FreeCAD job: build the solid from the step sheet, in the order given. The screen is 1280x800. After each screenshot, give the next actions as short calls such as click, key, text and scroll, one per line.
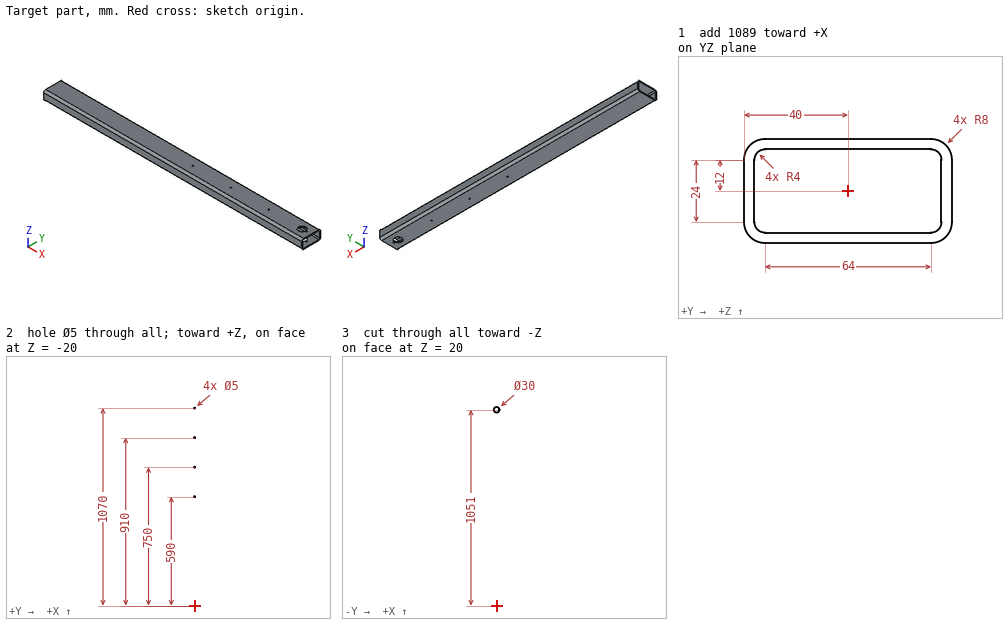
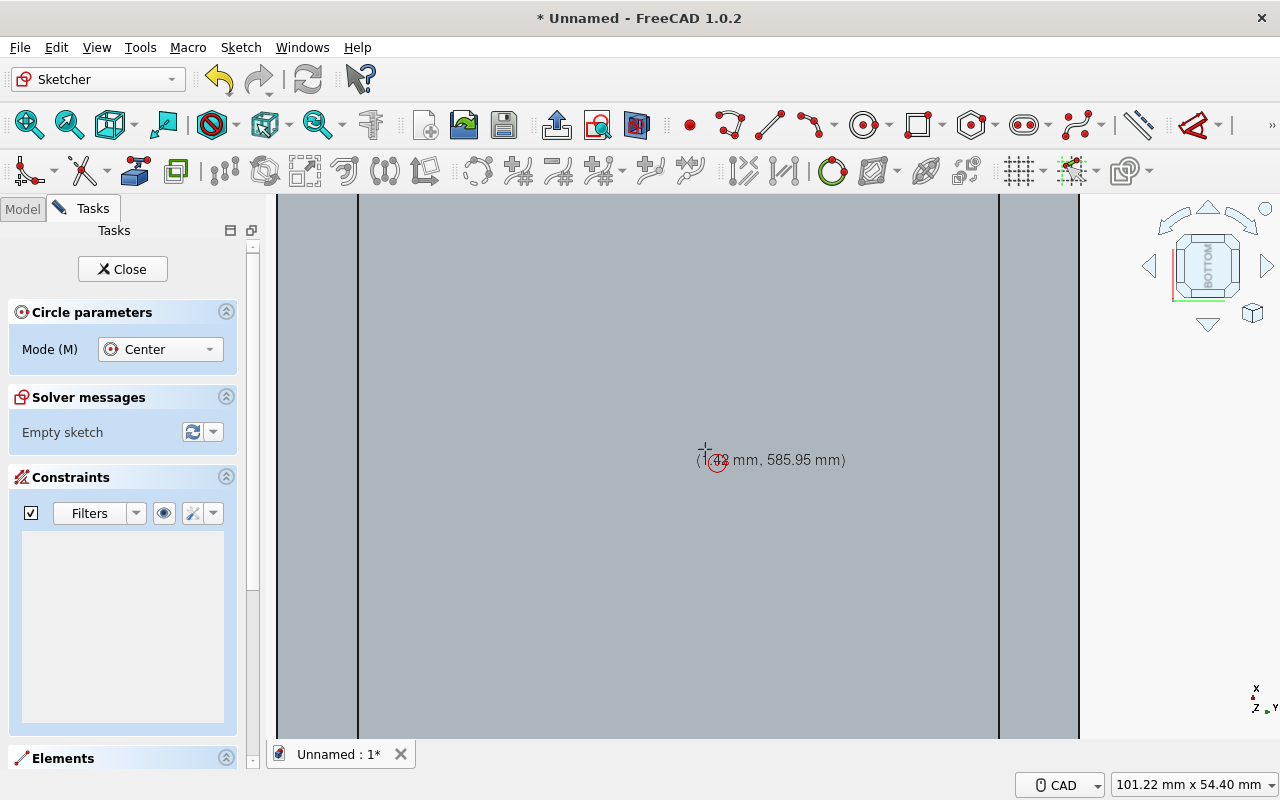
scroll(706, 445, down, 16)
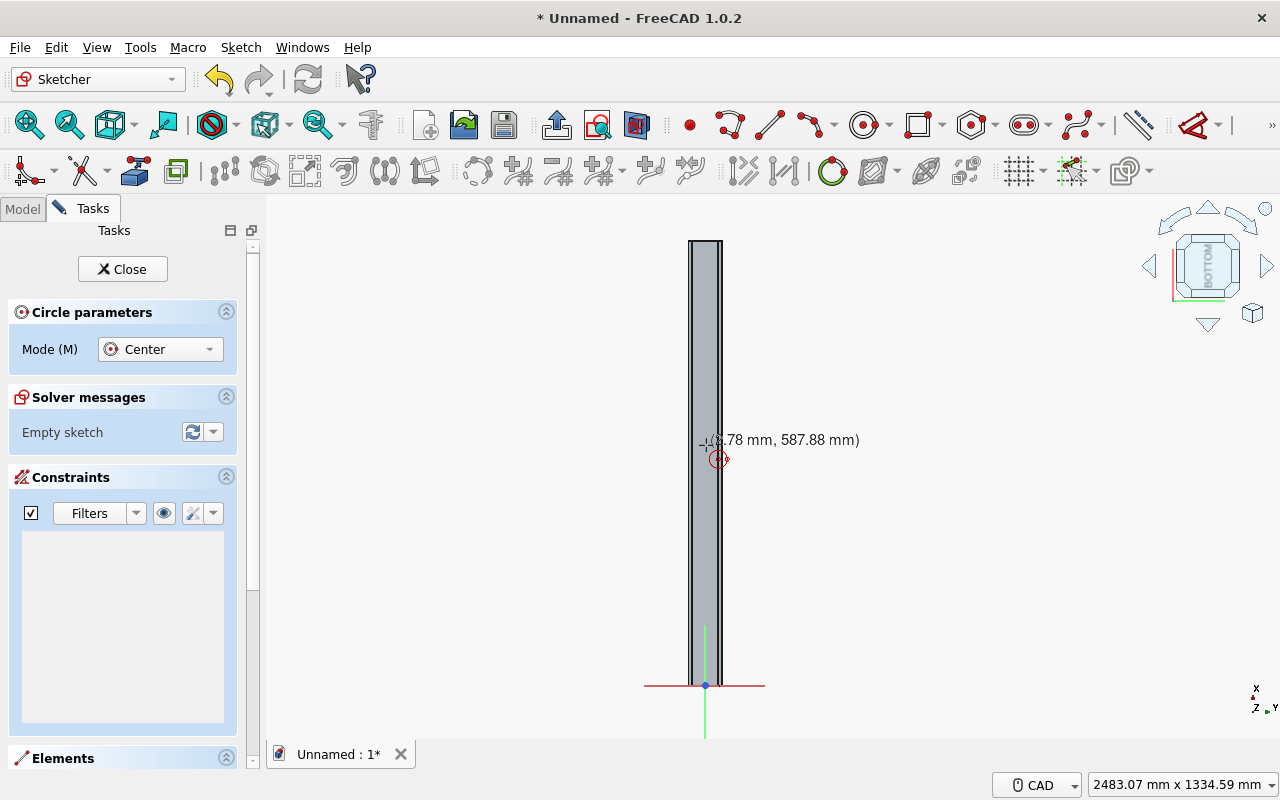
click(705, 445)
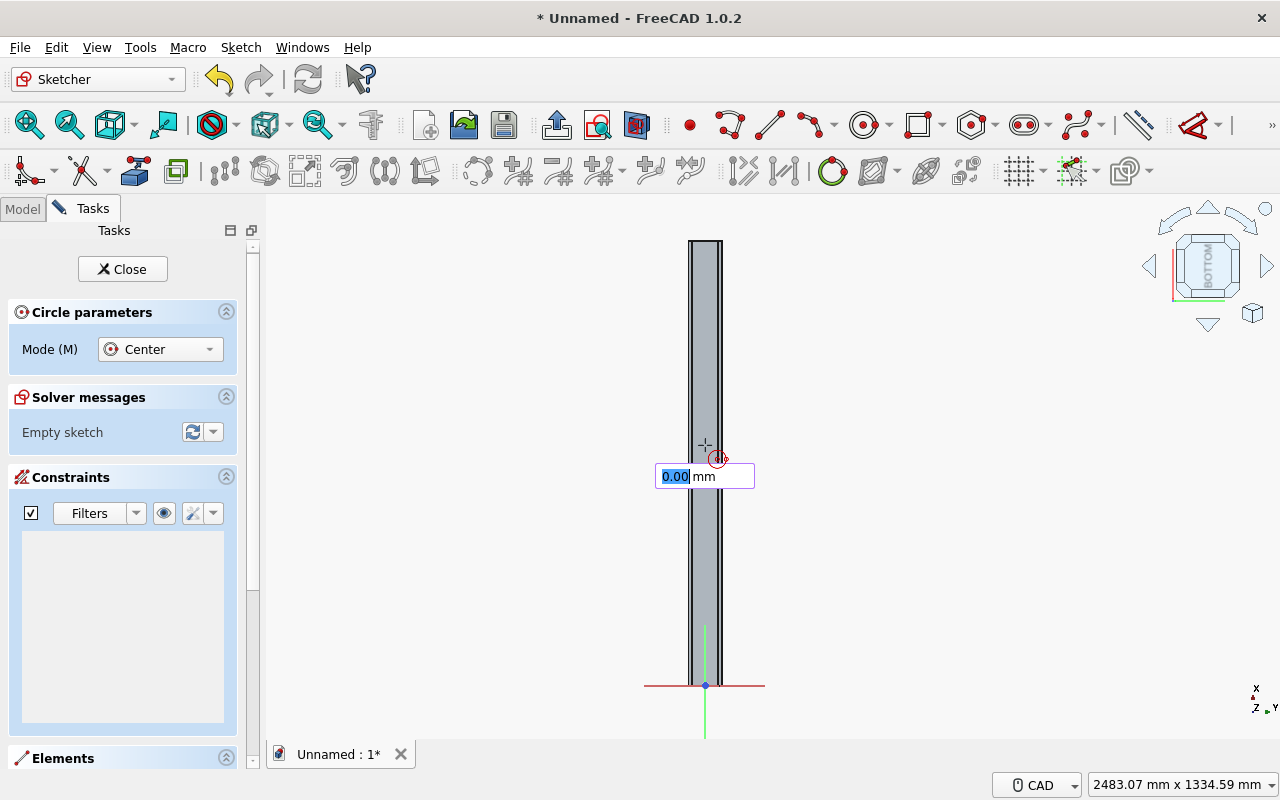
scroll(706, 444, up, 15)
move(703, 441)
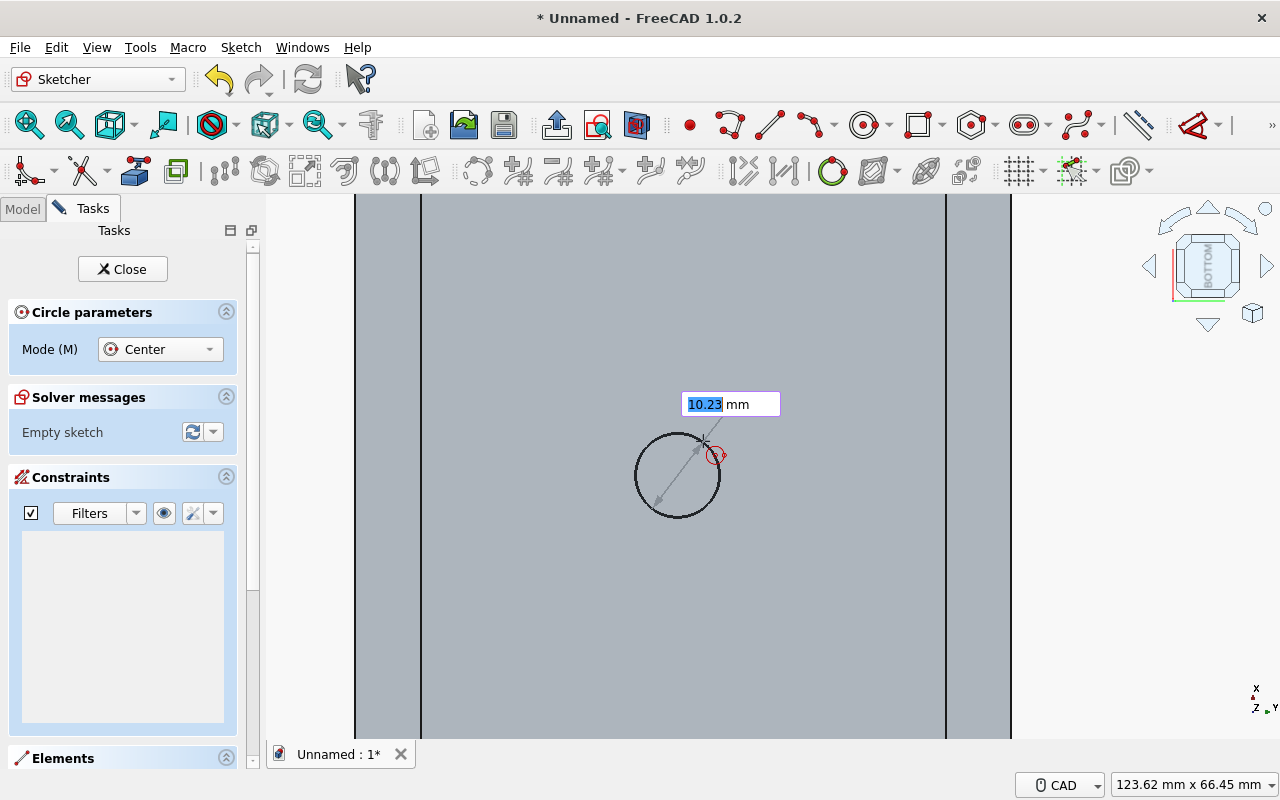
text(5)
key(Return)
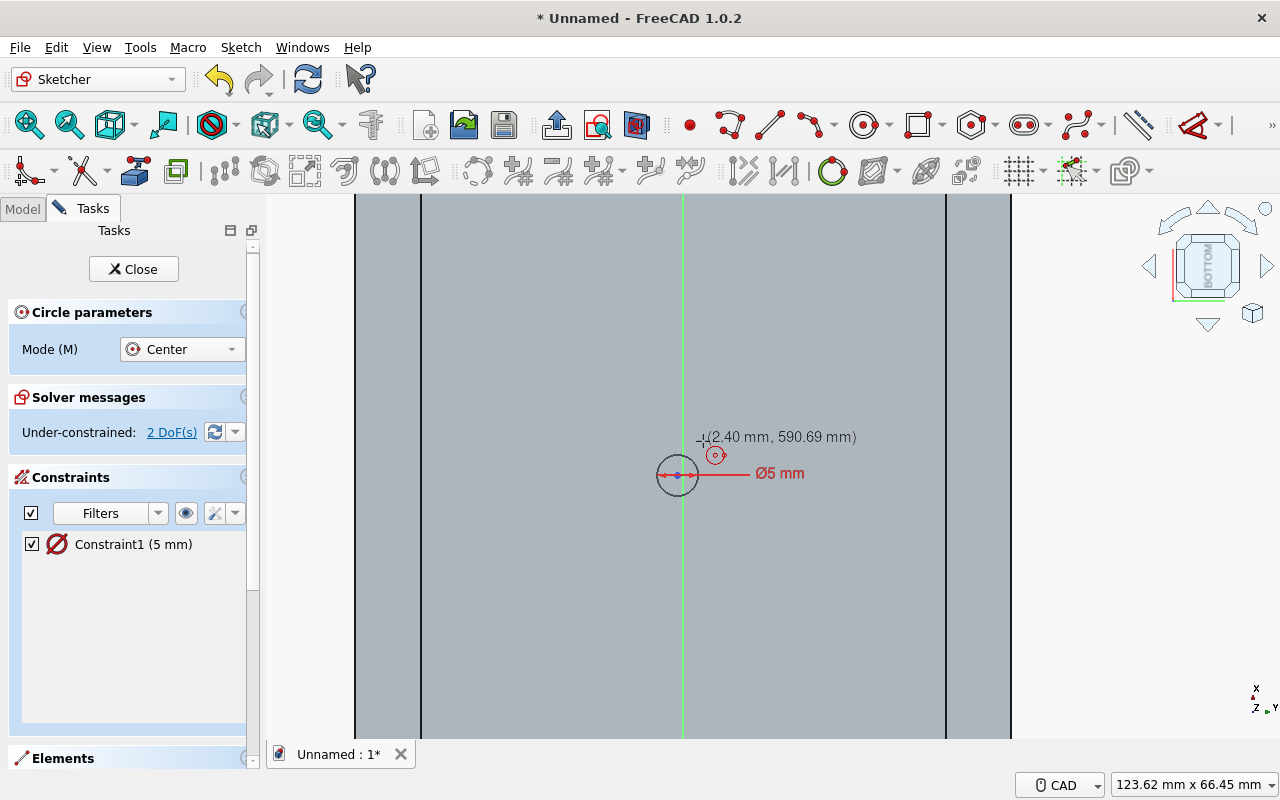
scroll(706, 444, down, 15)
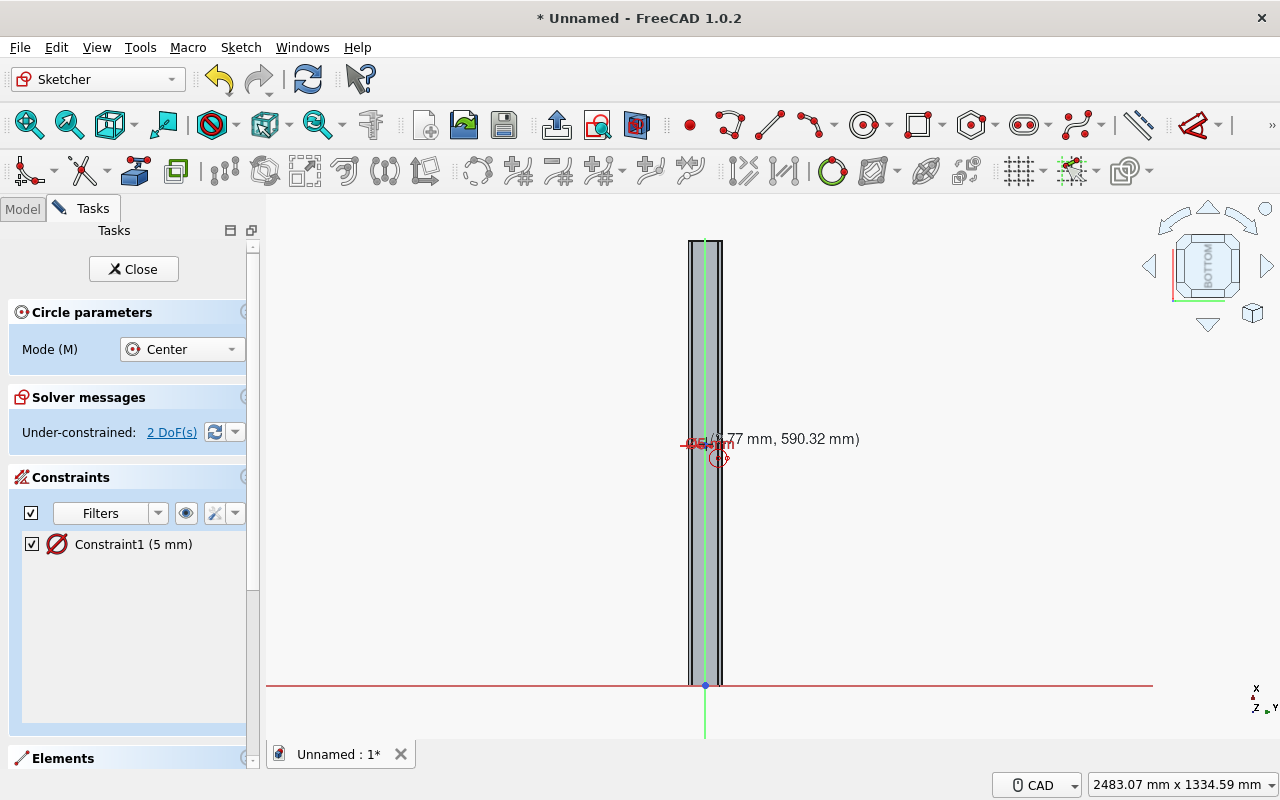
scroll(705, 379, up, 16)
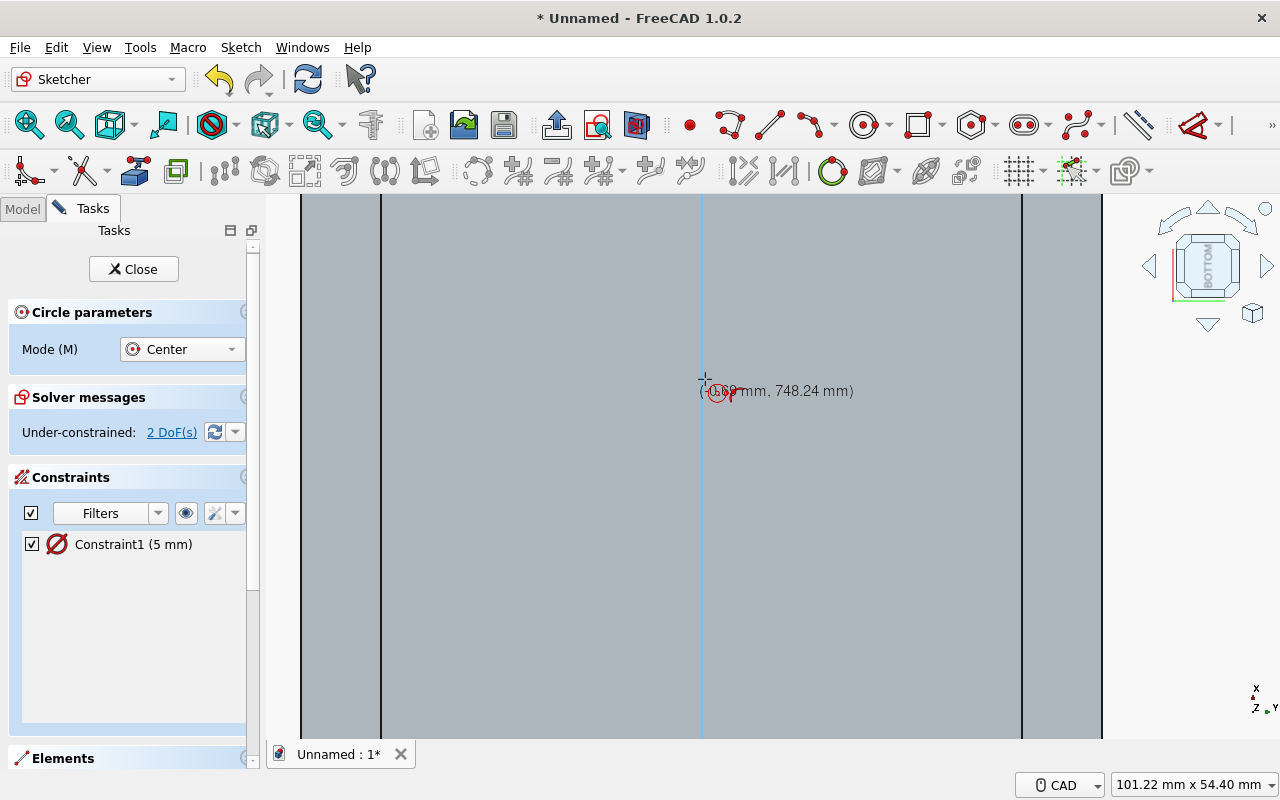
scroll(705, 379, down, 16)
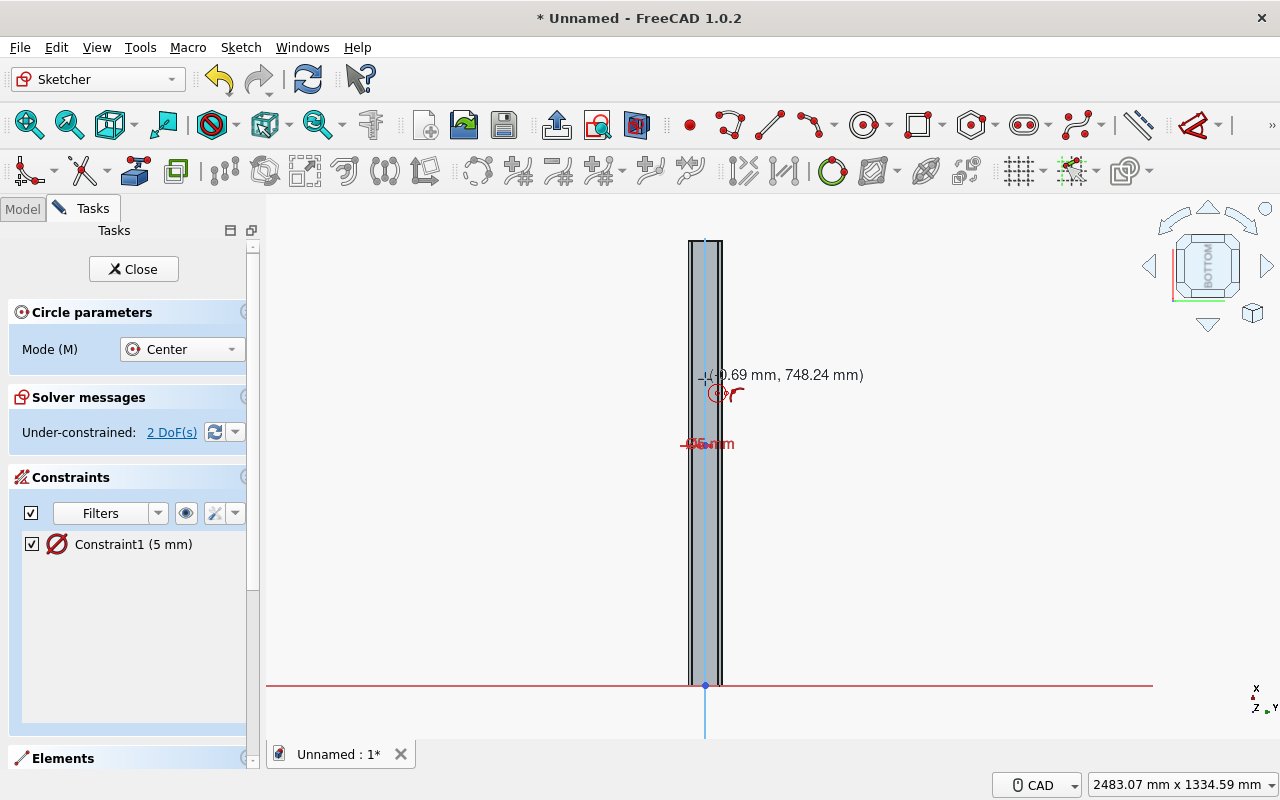
click(705, 379)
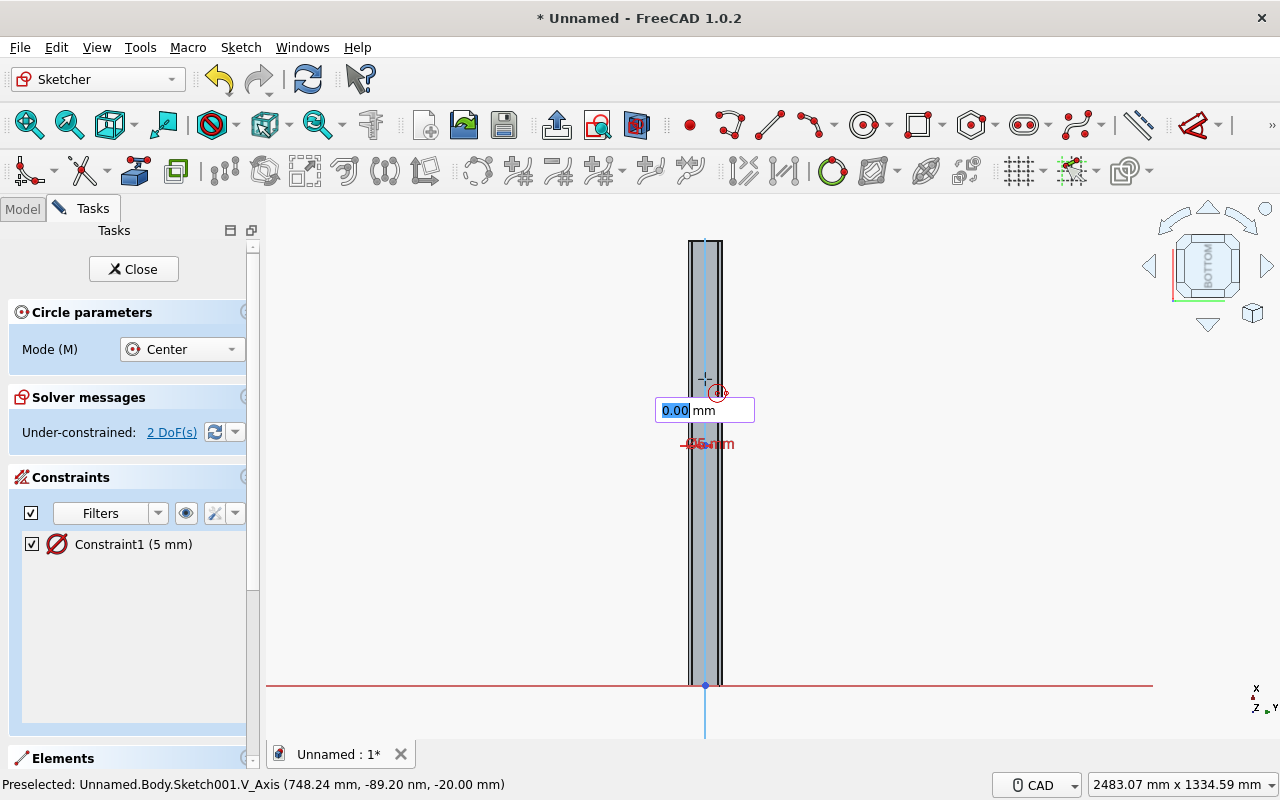
scroll(706, 379, up, 15)
move(703, 371)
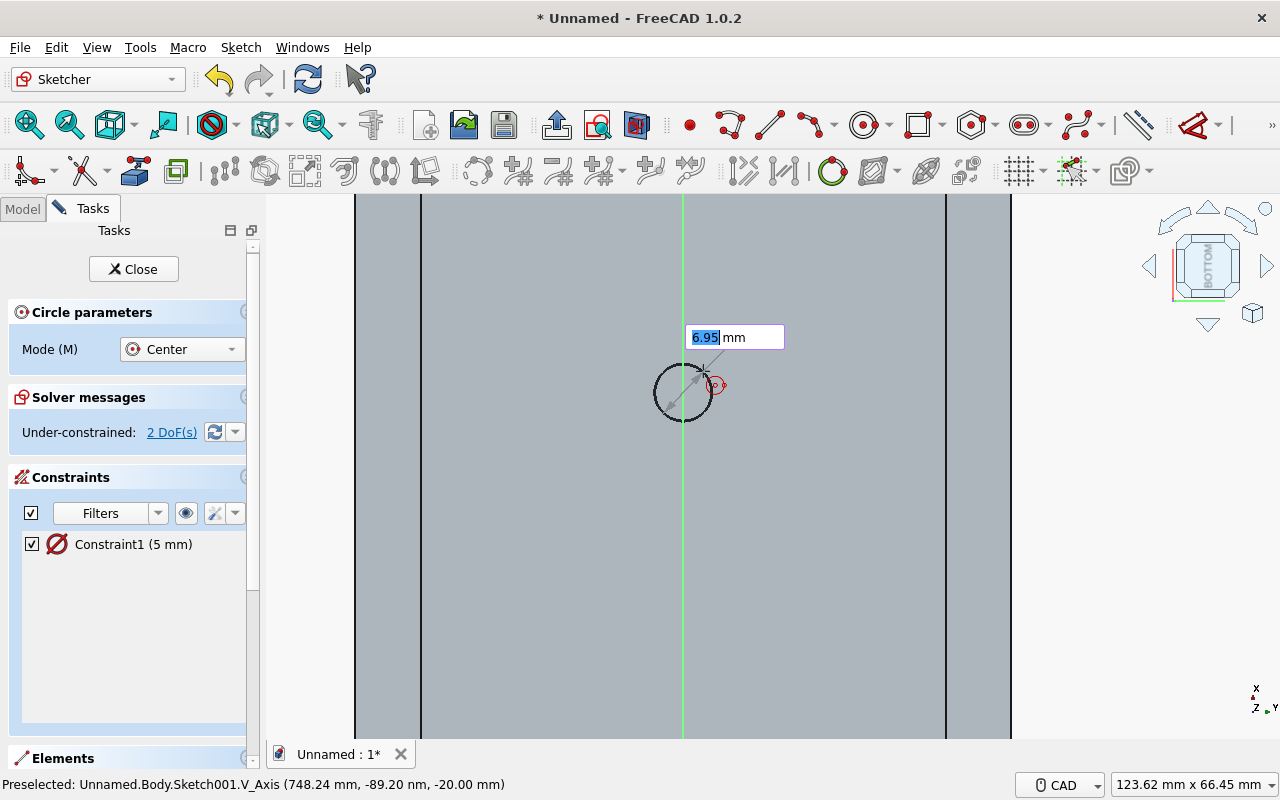
text(5)
key(Return)